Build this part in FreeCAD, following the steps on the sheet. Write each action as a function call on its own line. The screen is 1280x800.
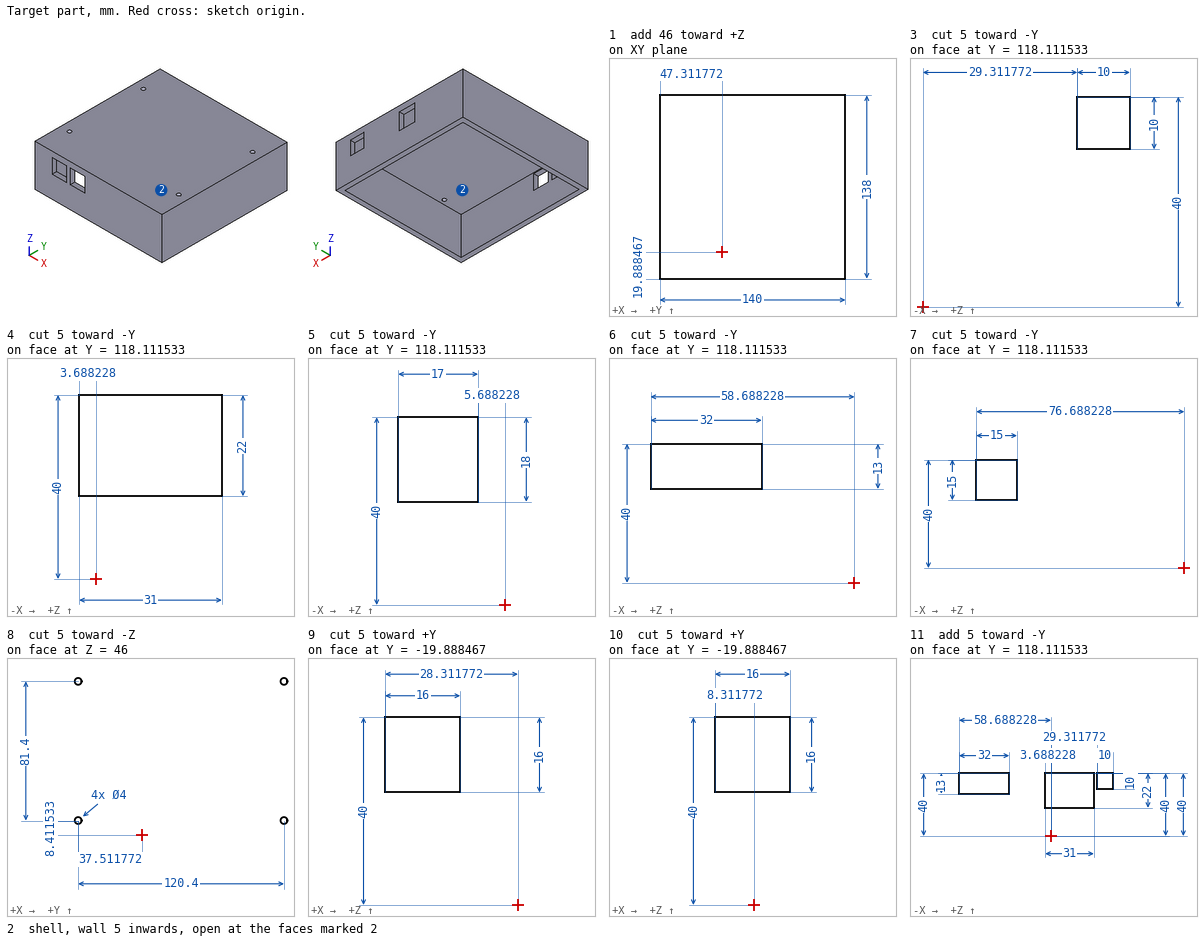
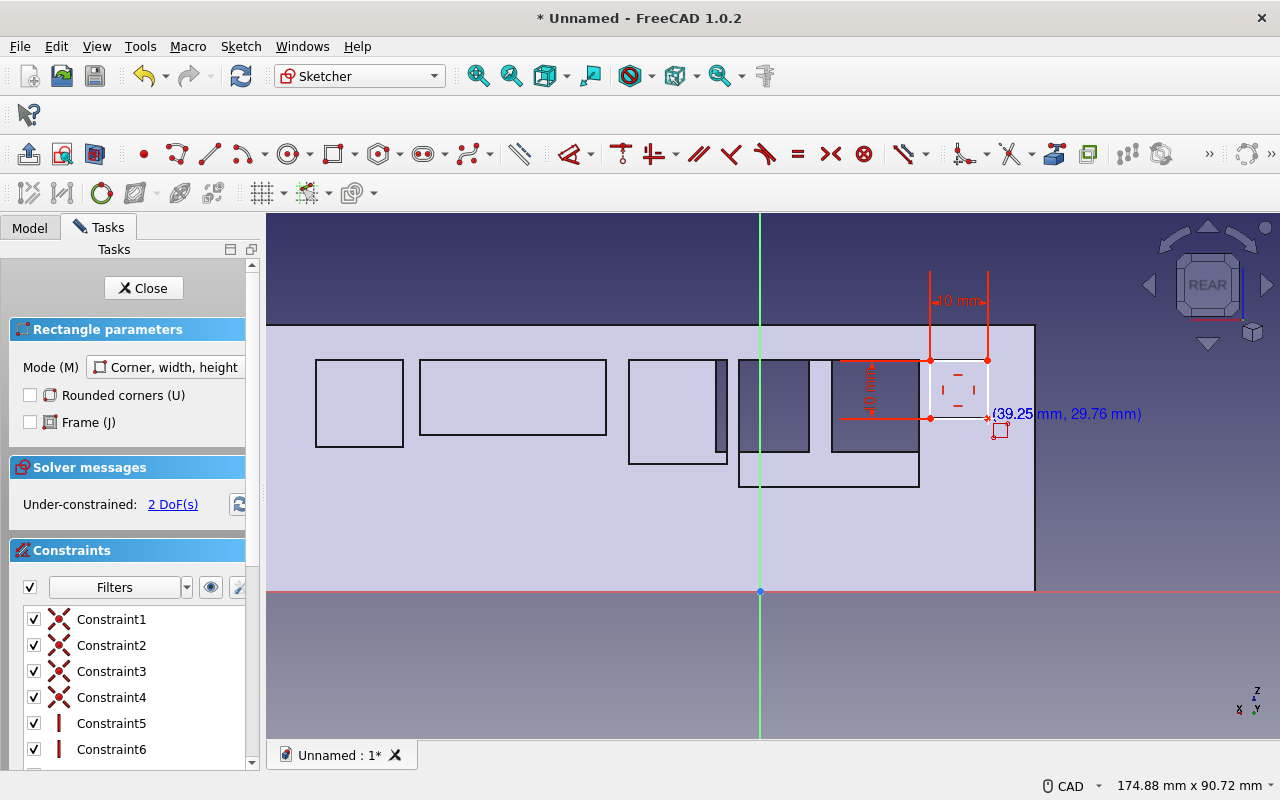
click(739, 360)
move(919, 487)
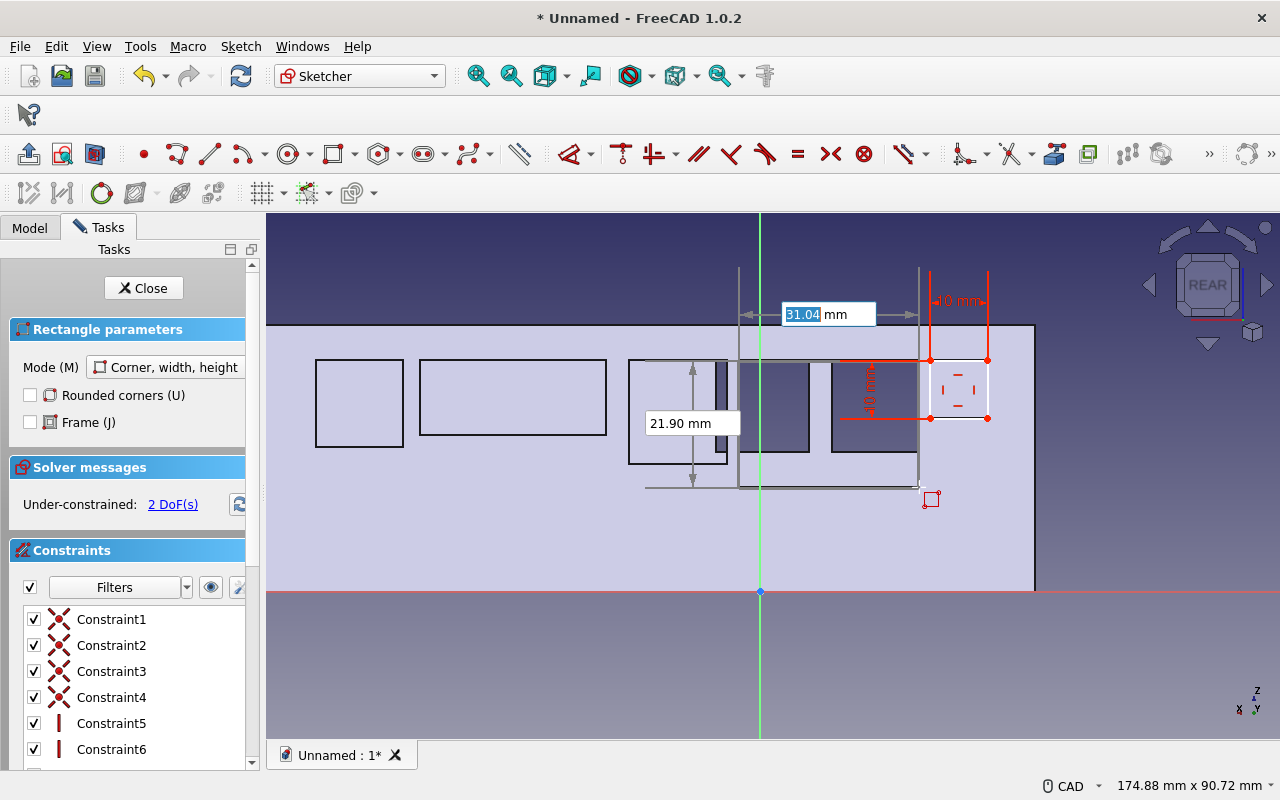
text(31)
key(Tab)
text(22)
key(Return)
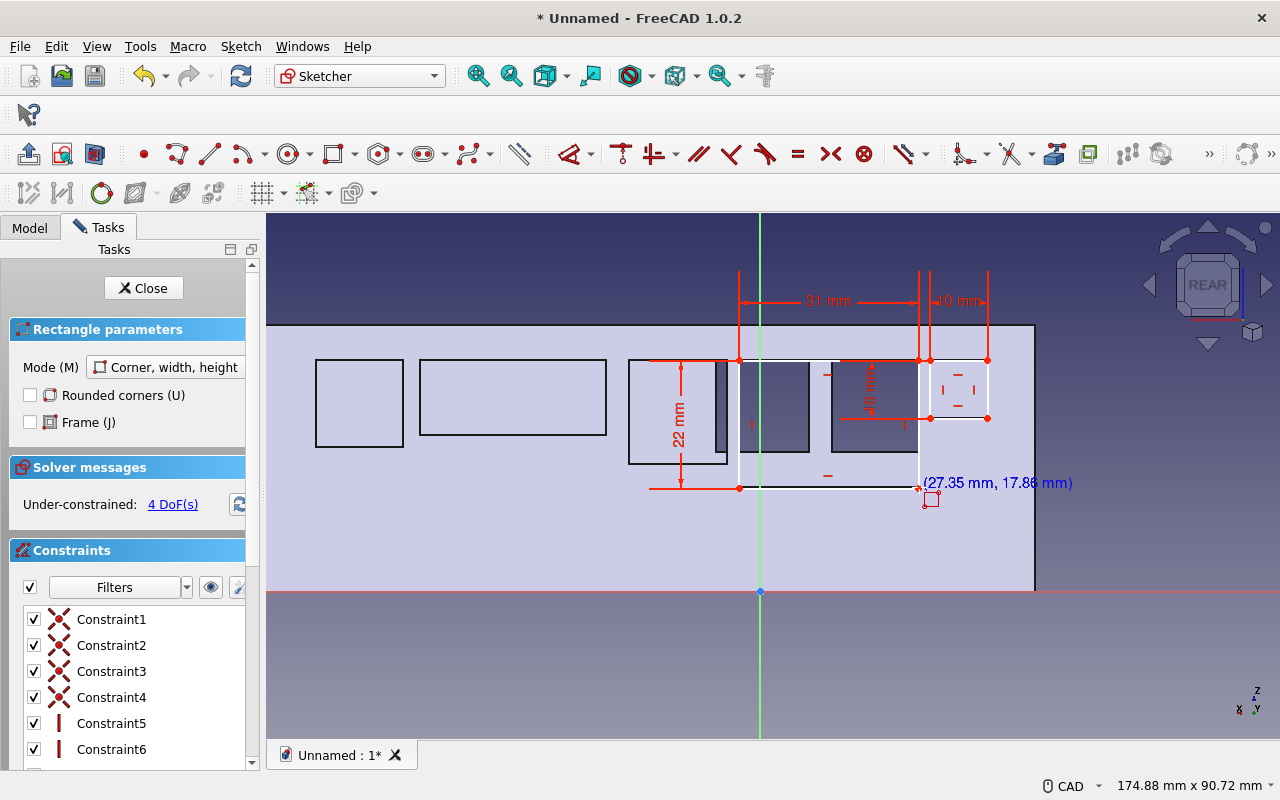
click(420, 360)
move(606, 435)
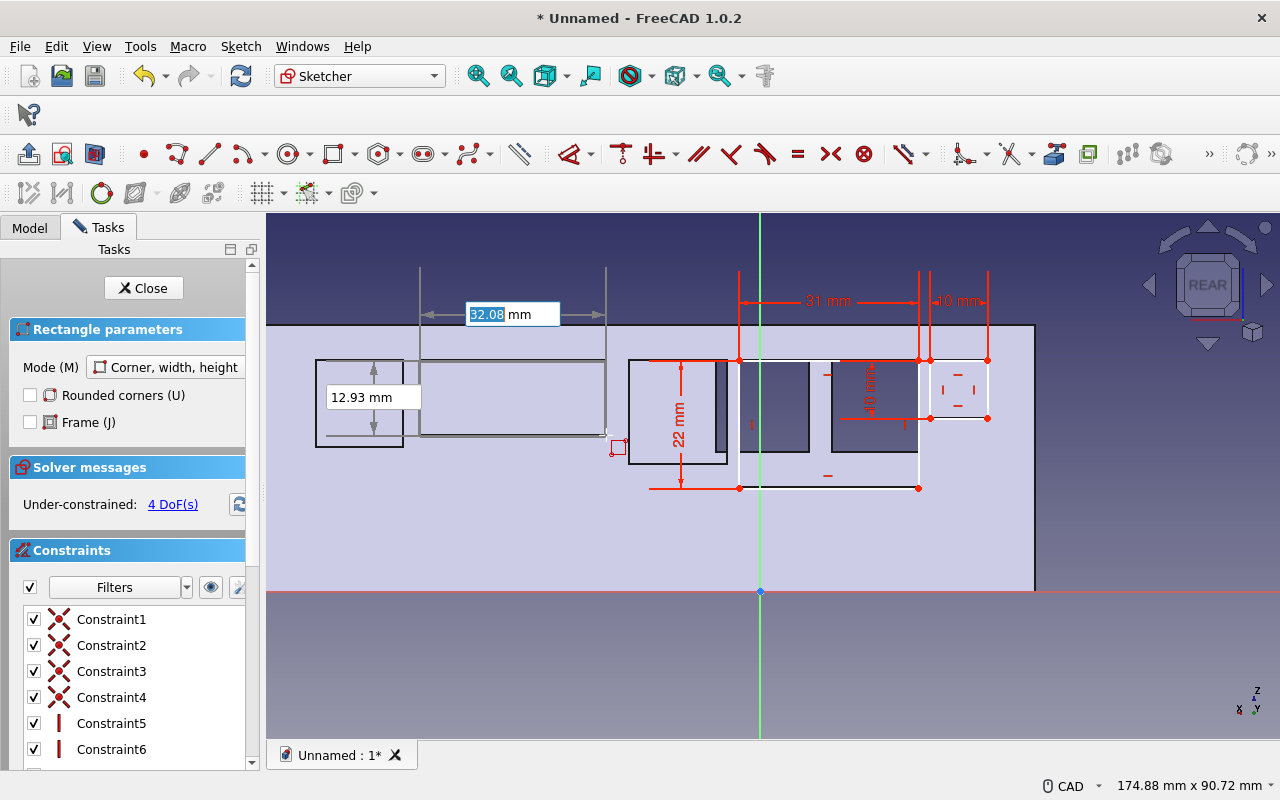
text(32)
key(Tab)
text(13)
key(Return)
key(Escape)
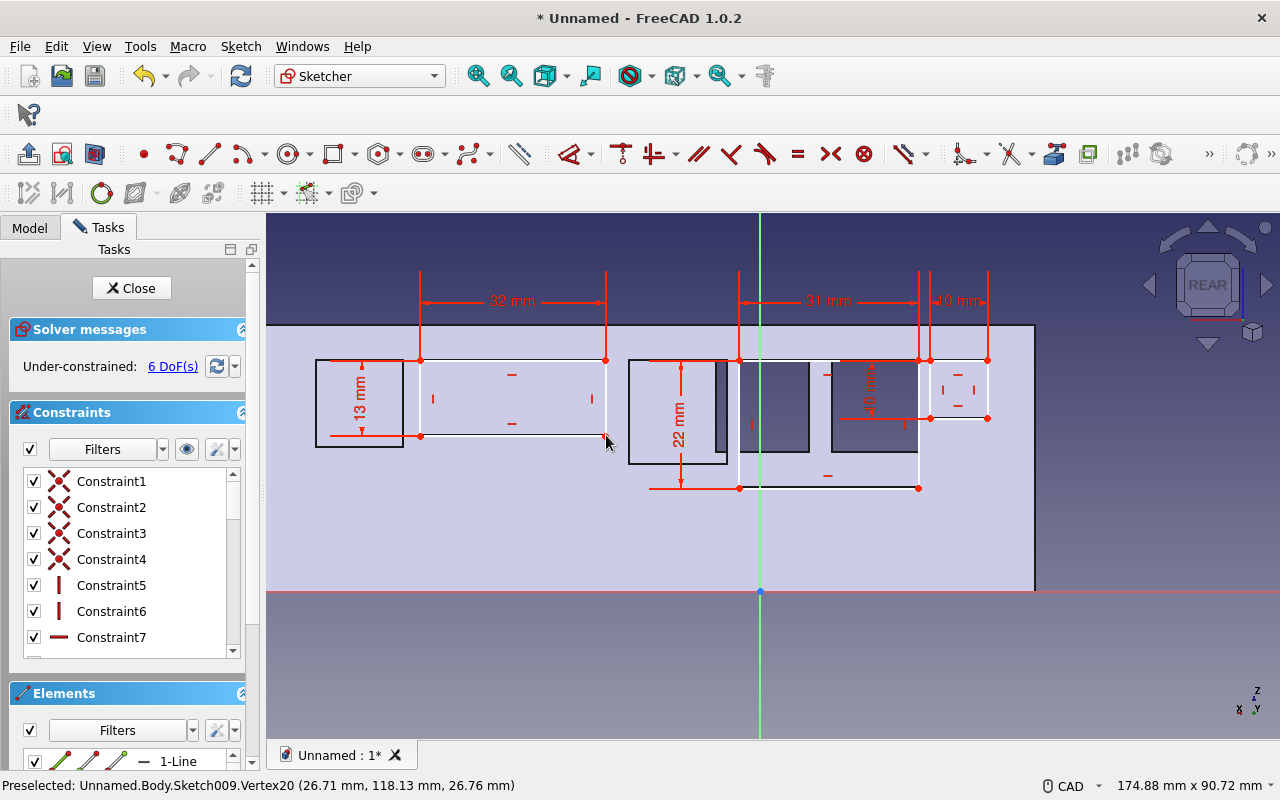
click(568, 154)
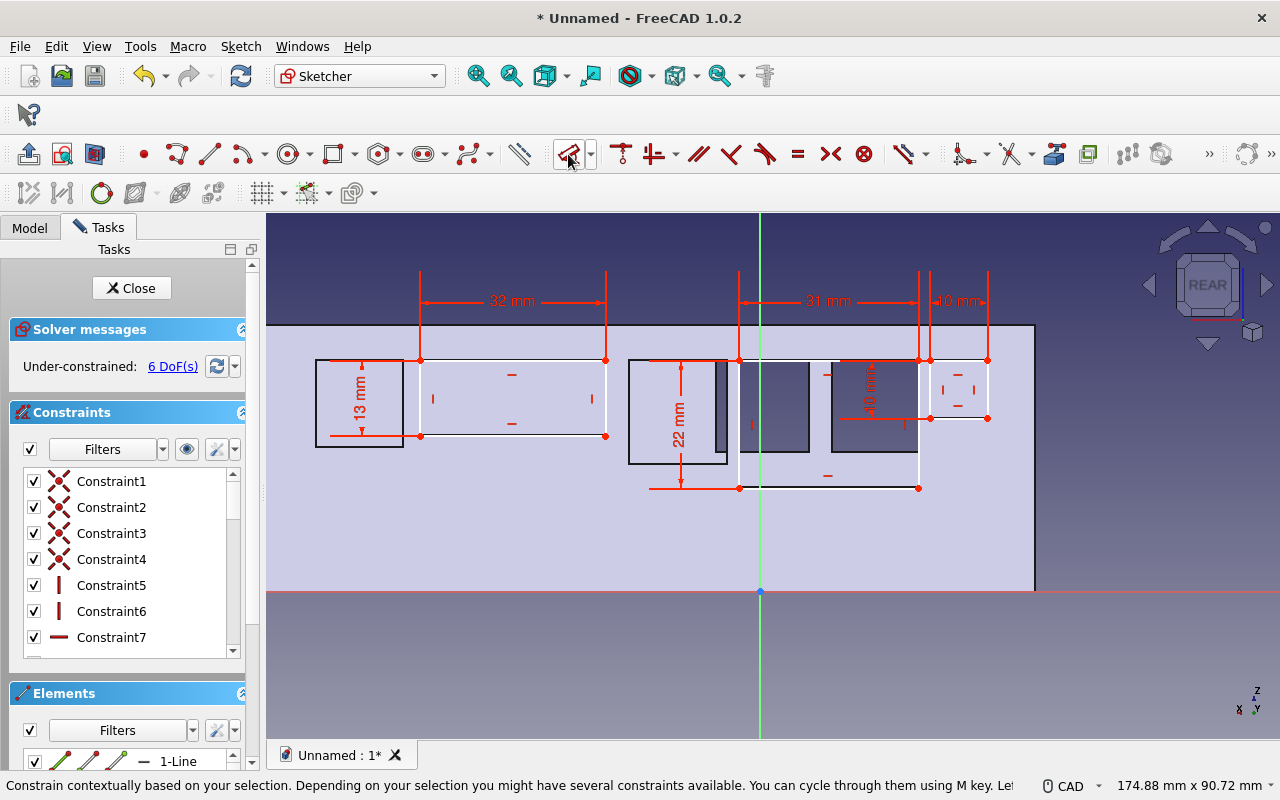
click(930, 361)
click(964, 476)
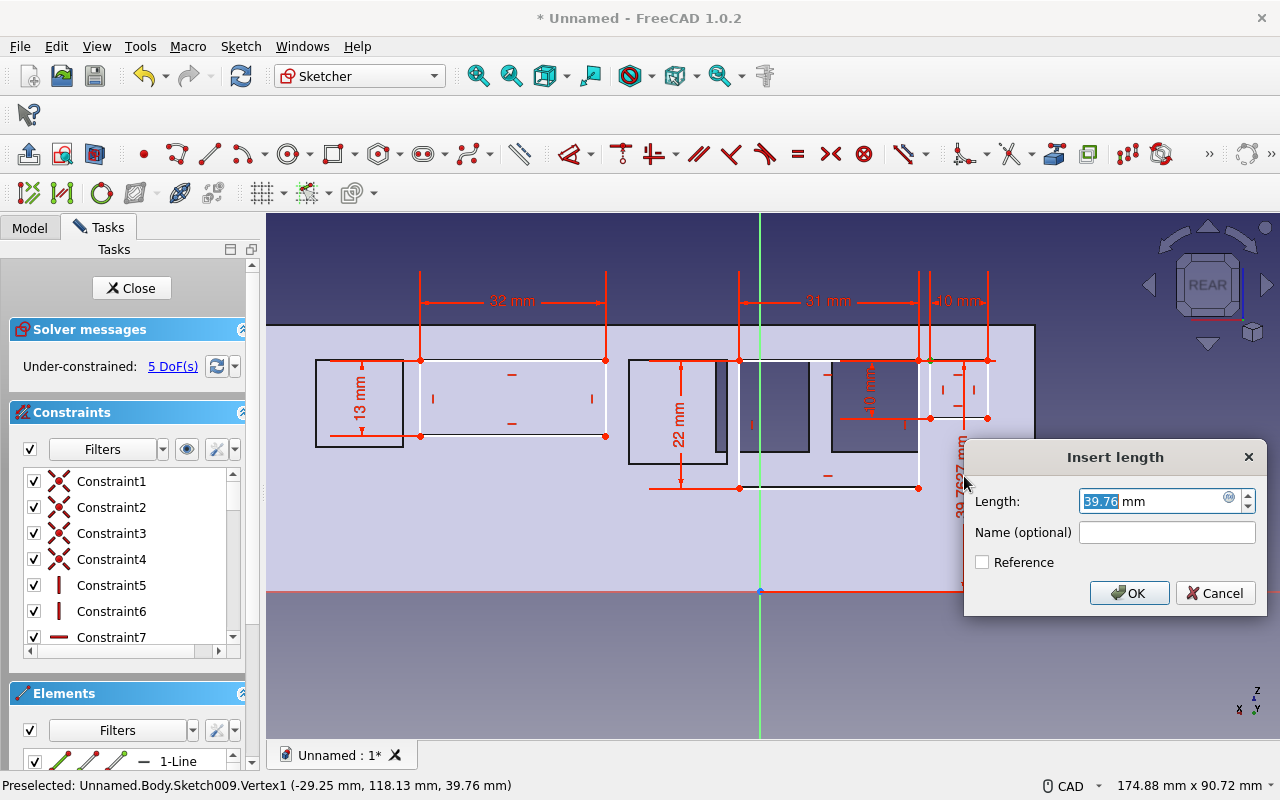
text(40)
key(Return)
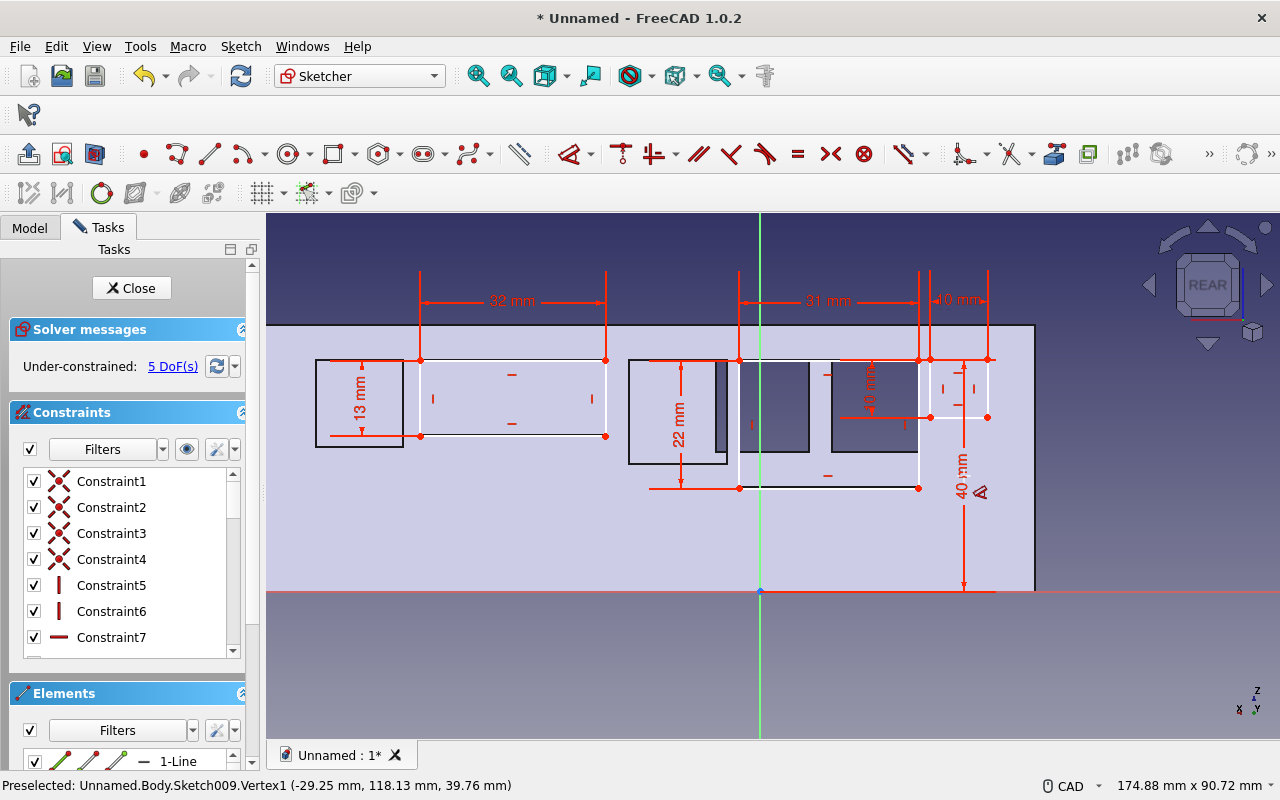
click(739, 361)
click(794, 423)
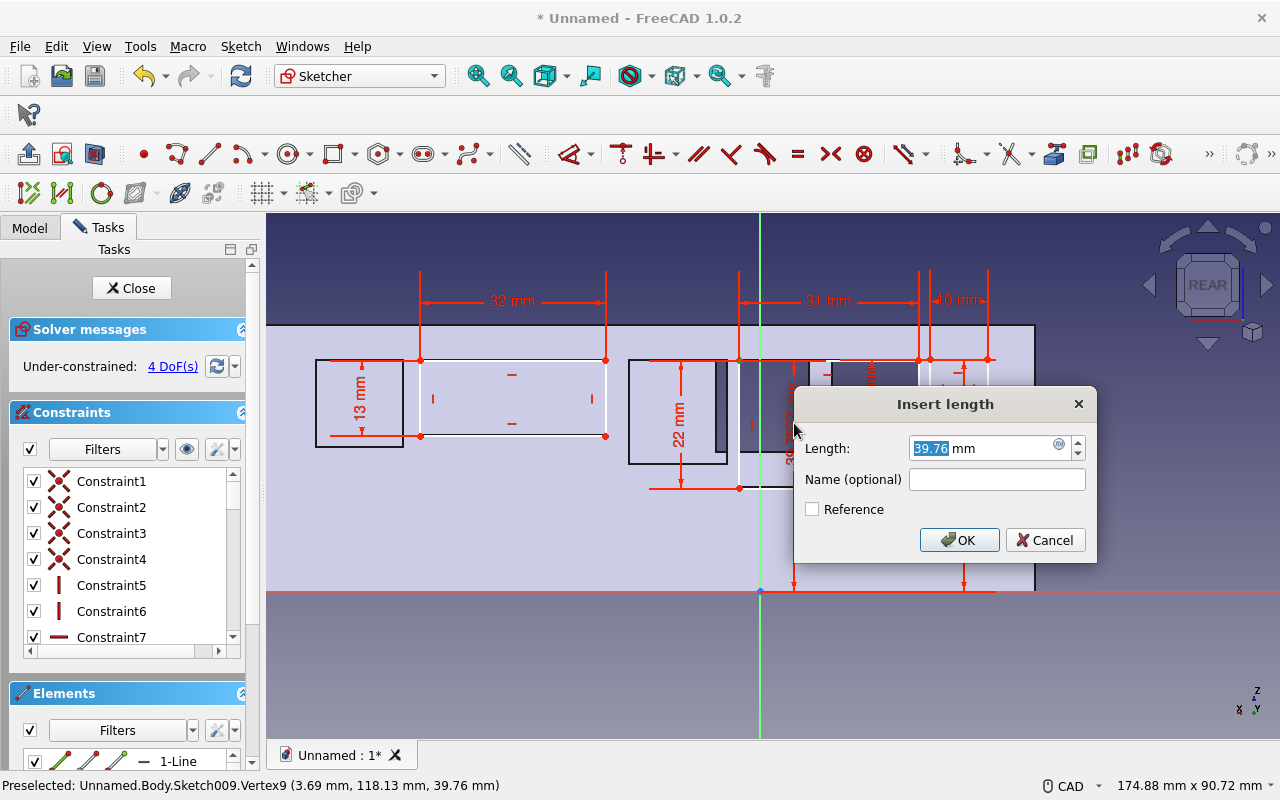
text(40)
key(Return)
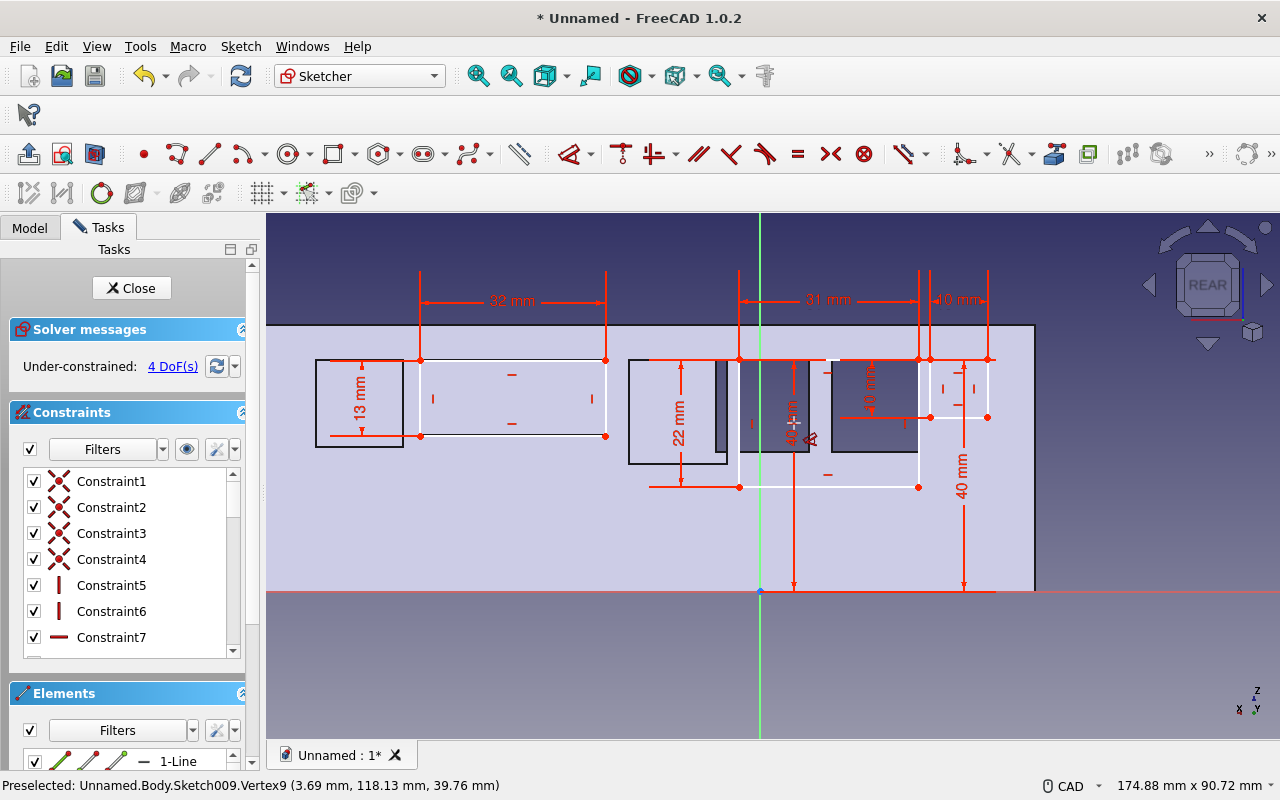
click(420, 361)
click(386, 476)